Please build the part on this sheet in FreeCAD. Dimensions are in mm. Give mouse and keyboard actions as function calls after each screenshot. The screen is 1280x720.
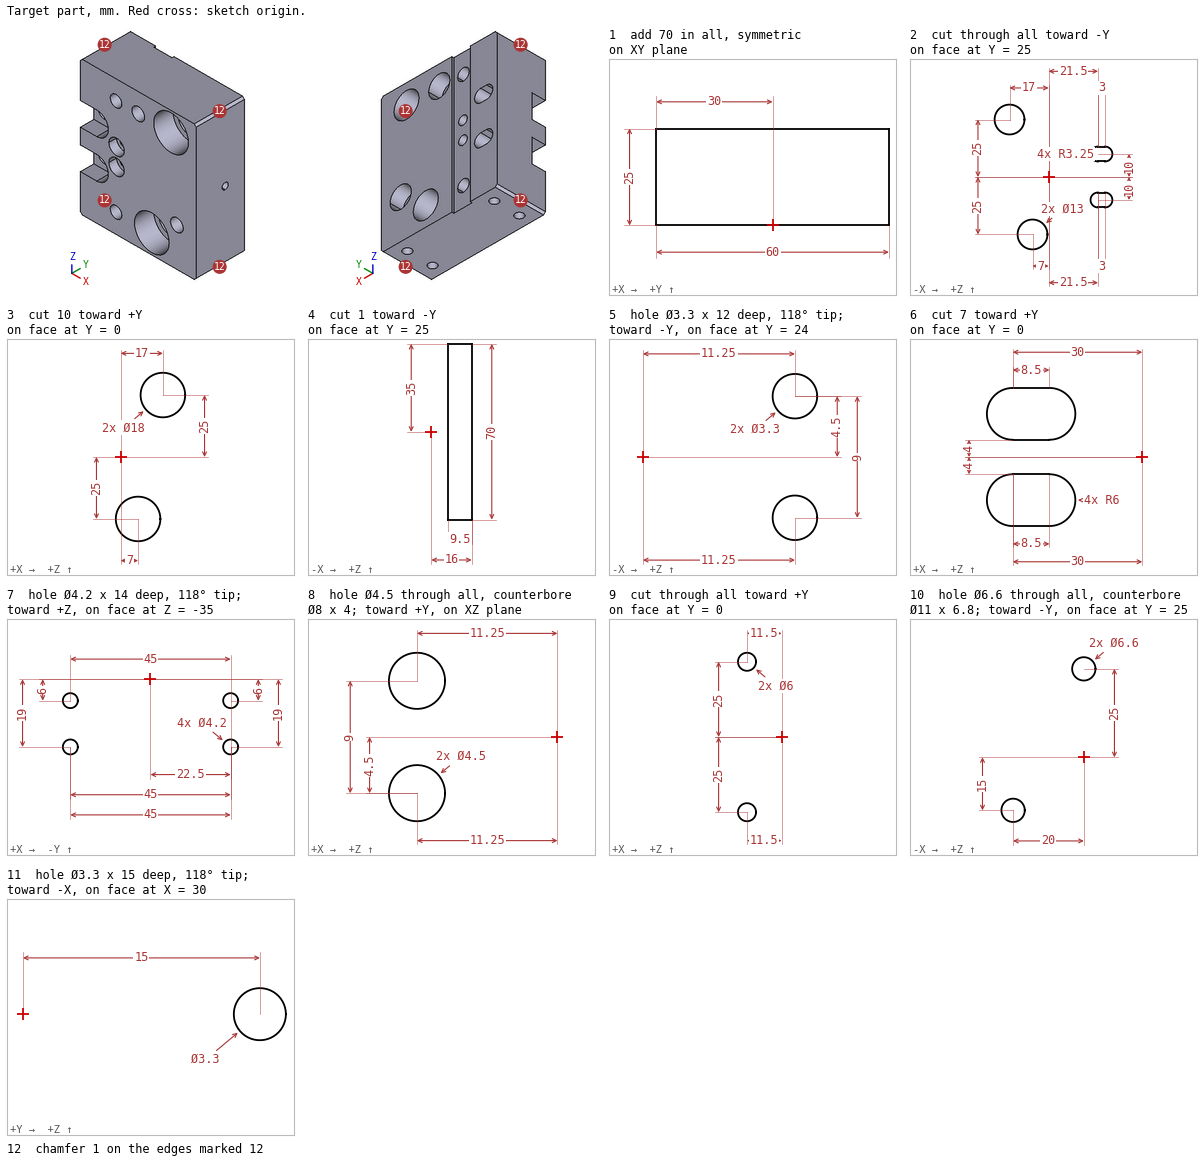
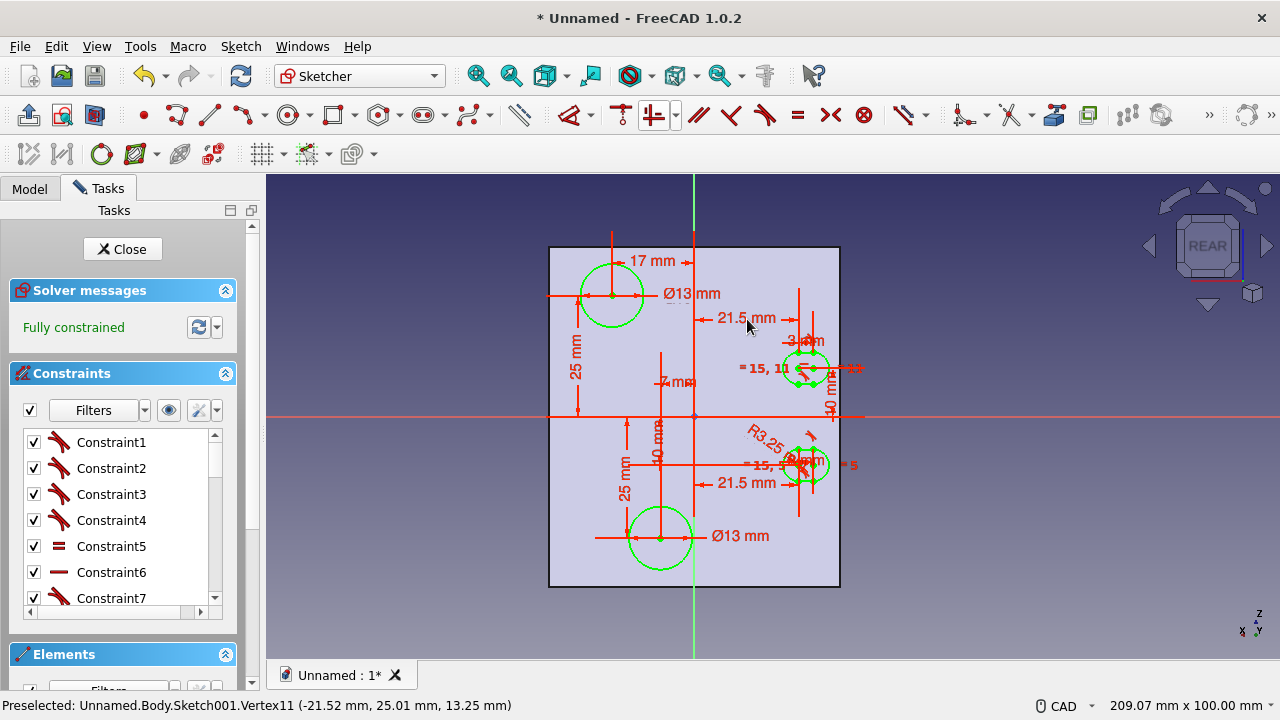
click(123, 249)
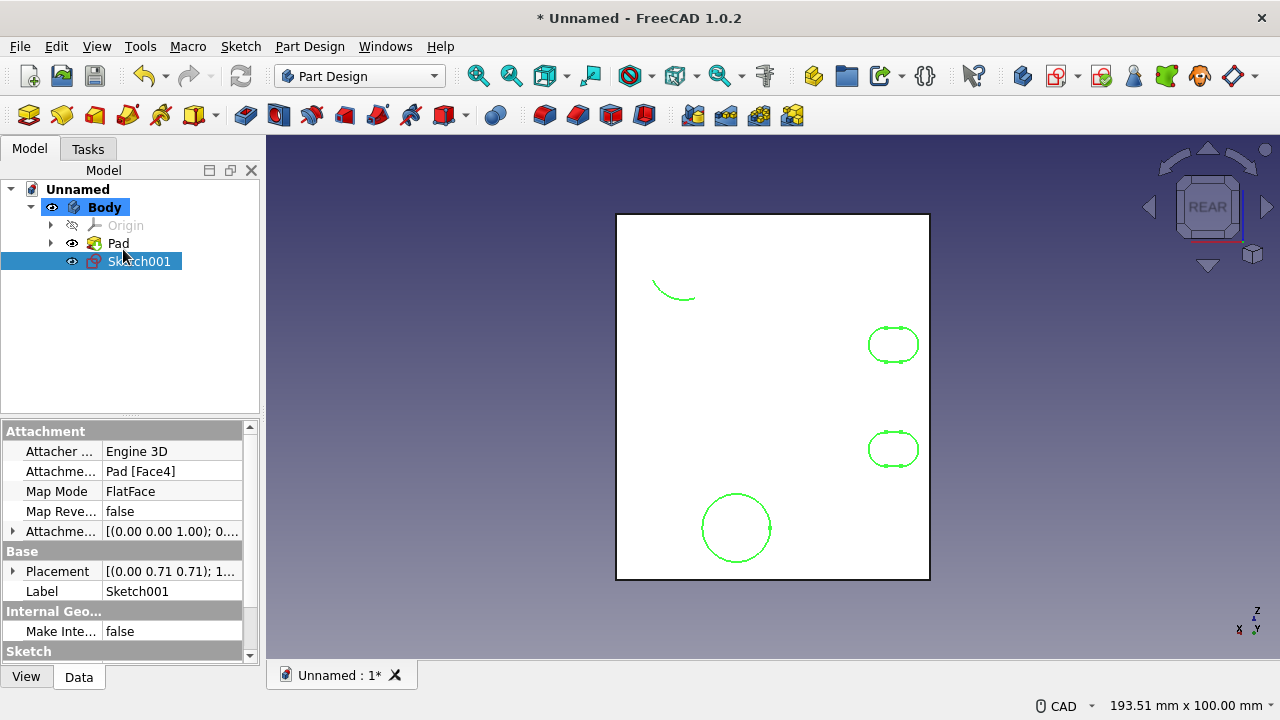
click(246, 116)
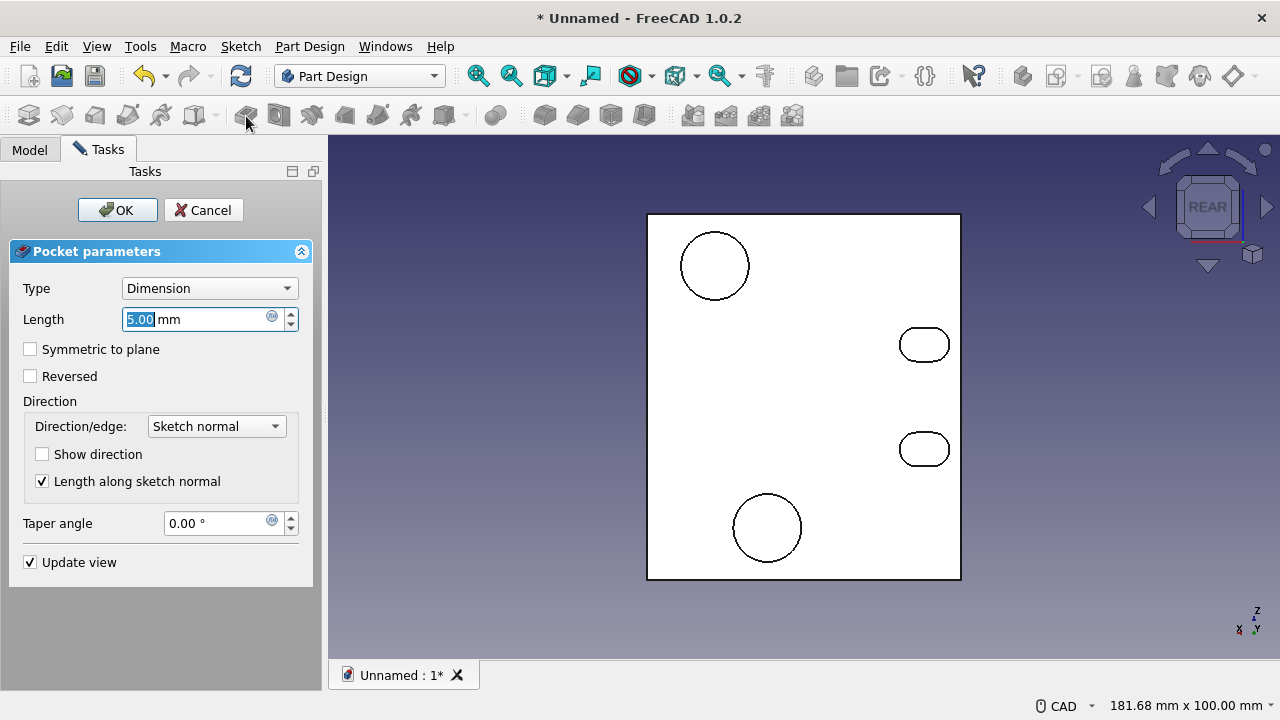
click(210, 288)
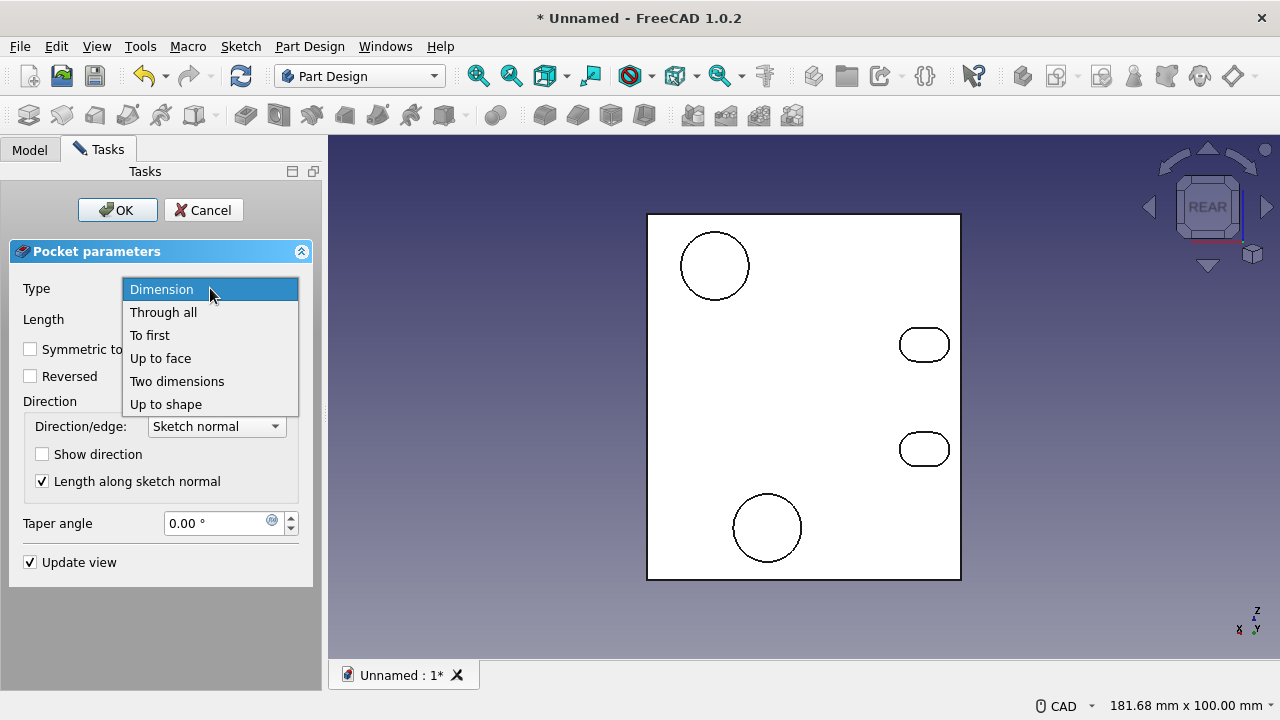
click(208, 312)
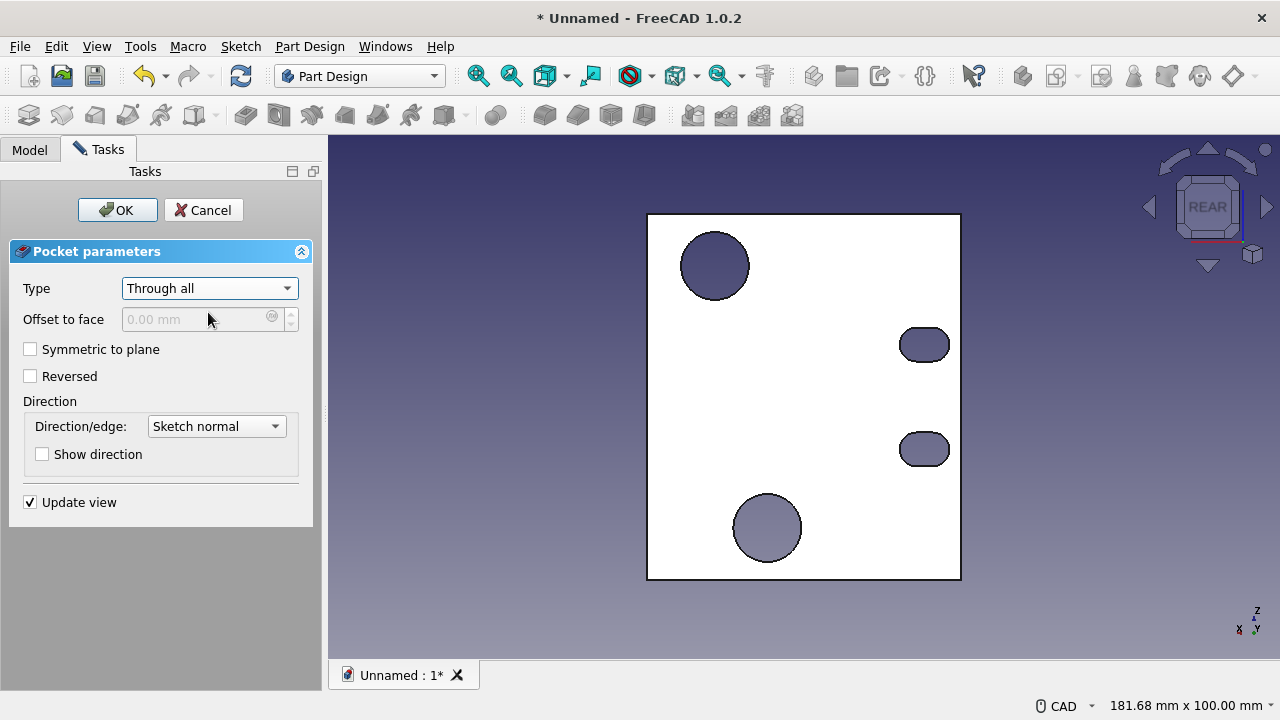
click(118, 210)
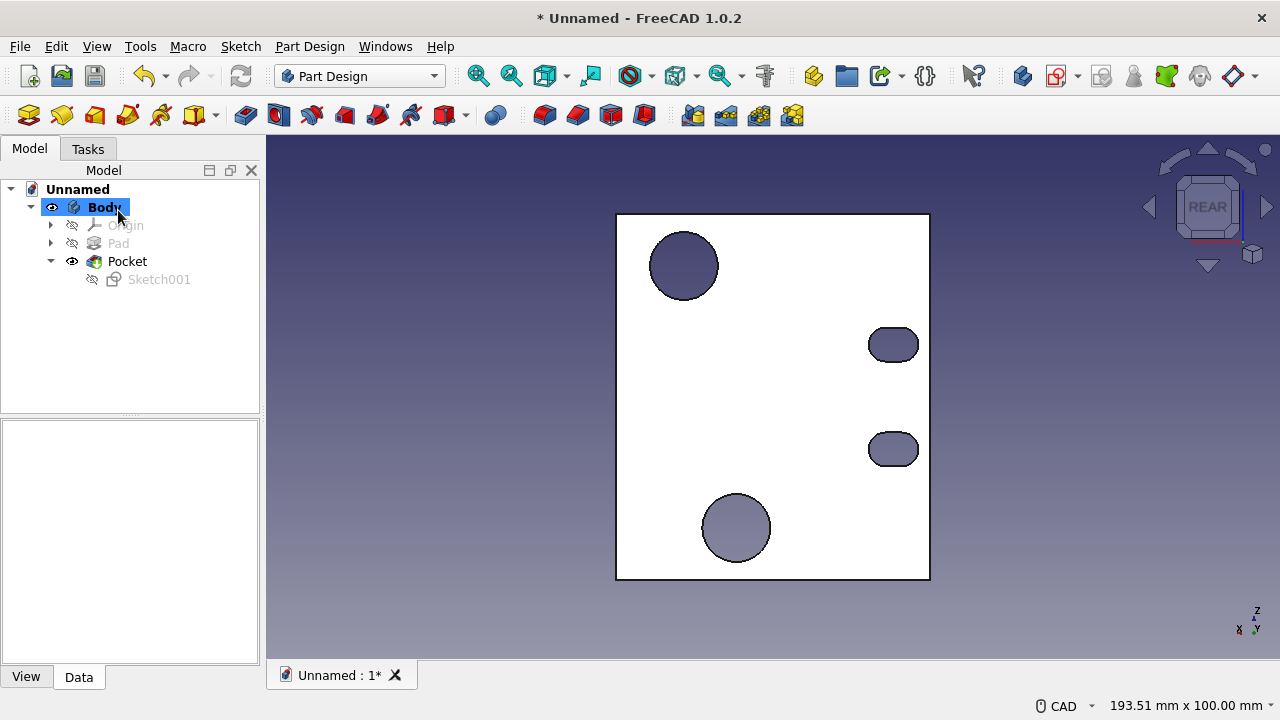
key(0)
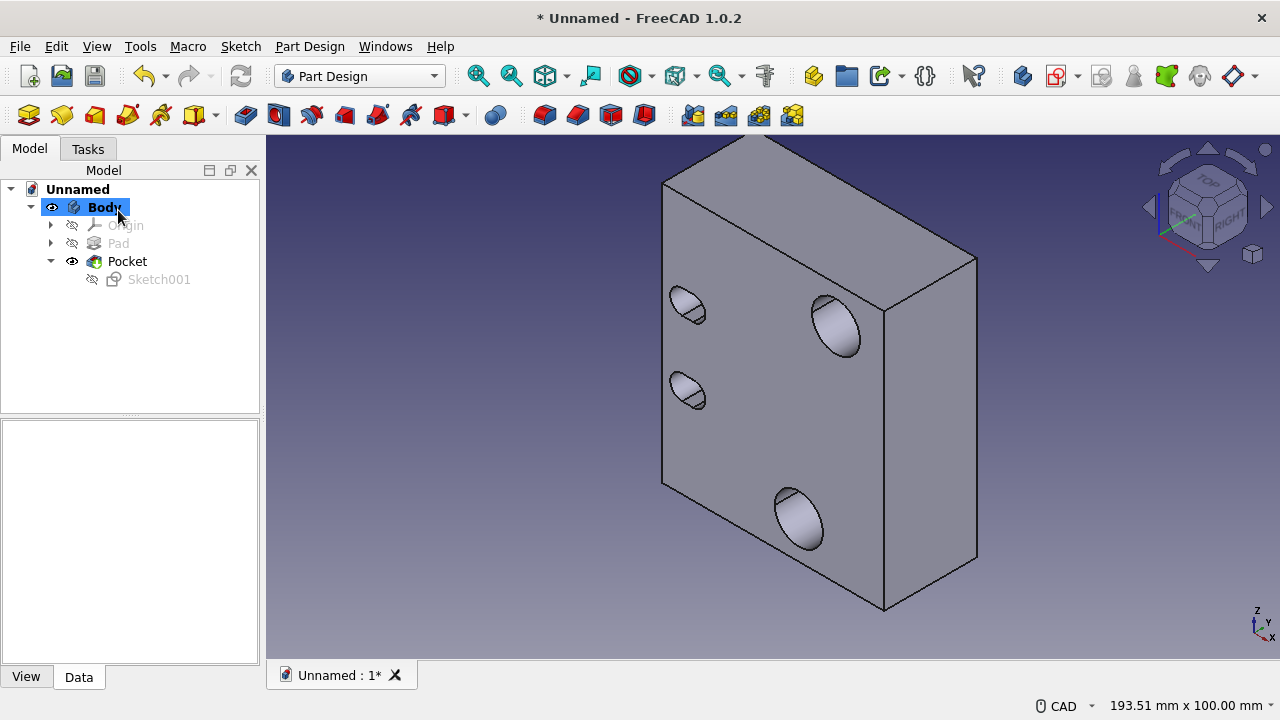
key(v)
key(f)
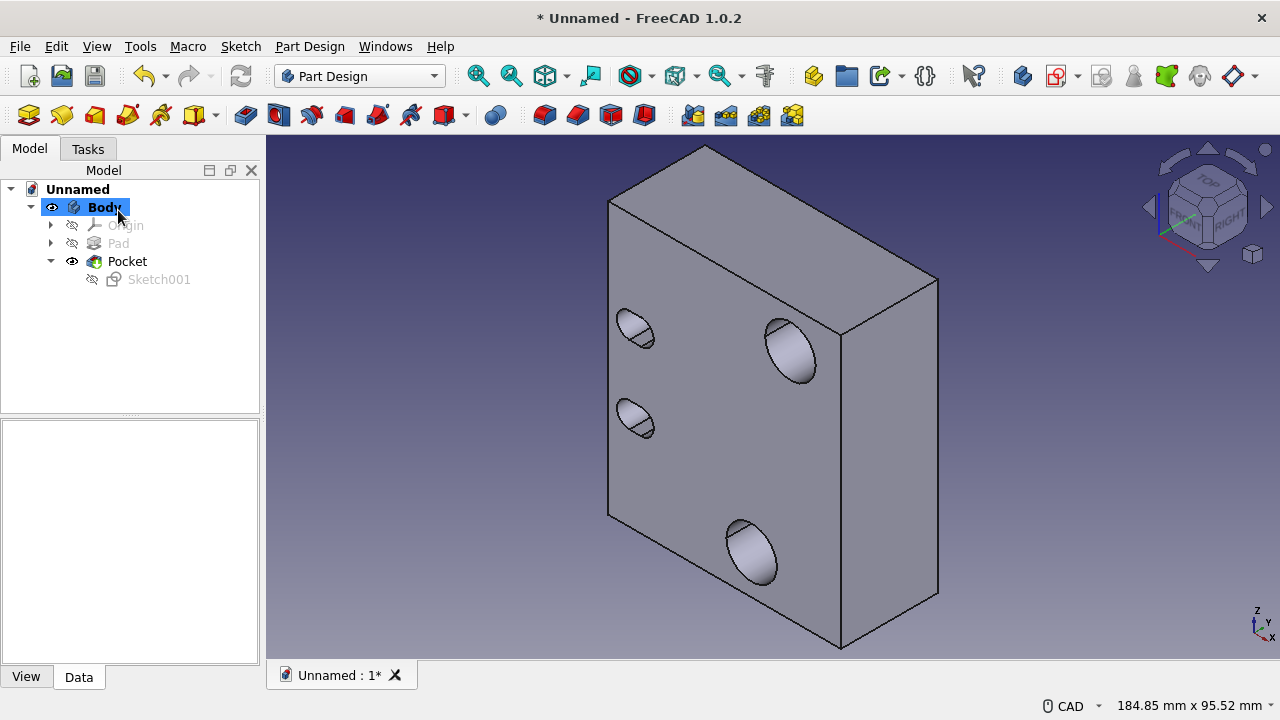
click(725, 424)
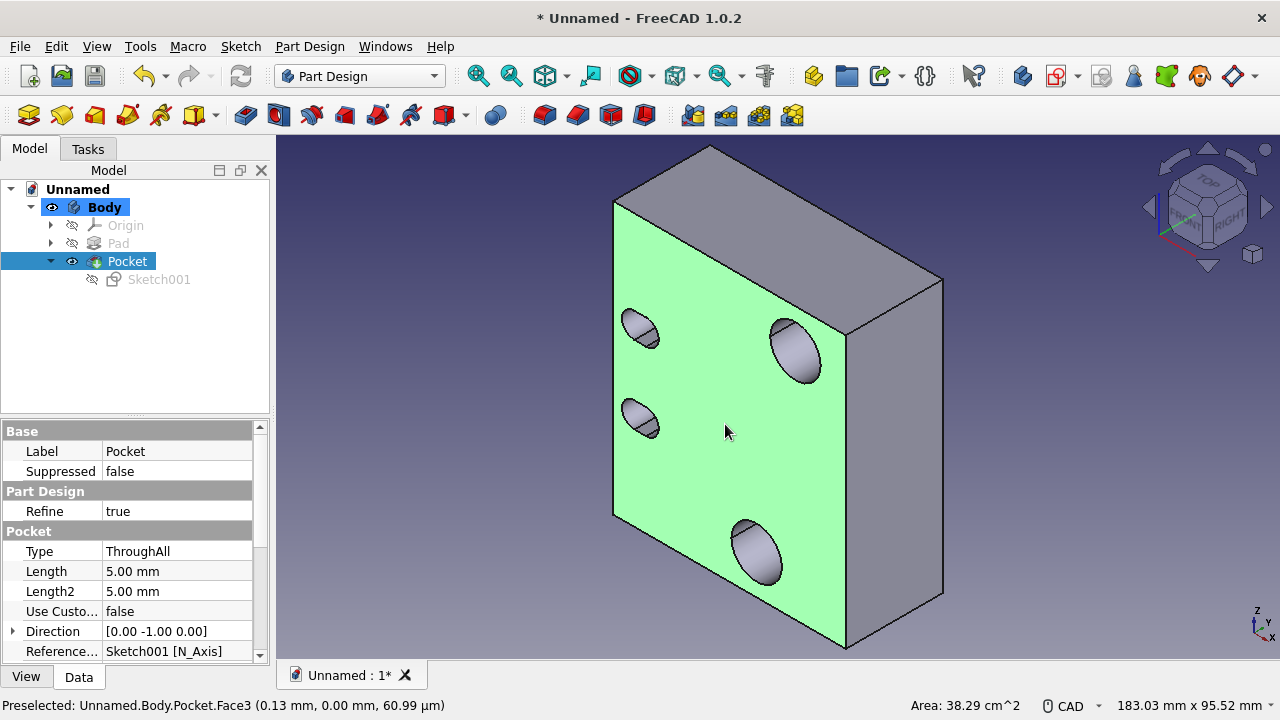
click(1056, 76)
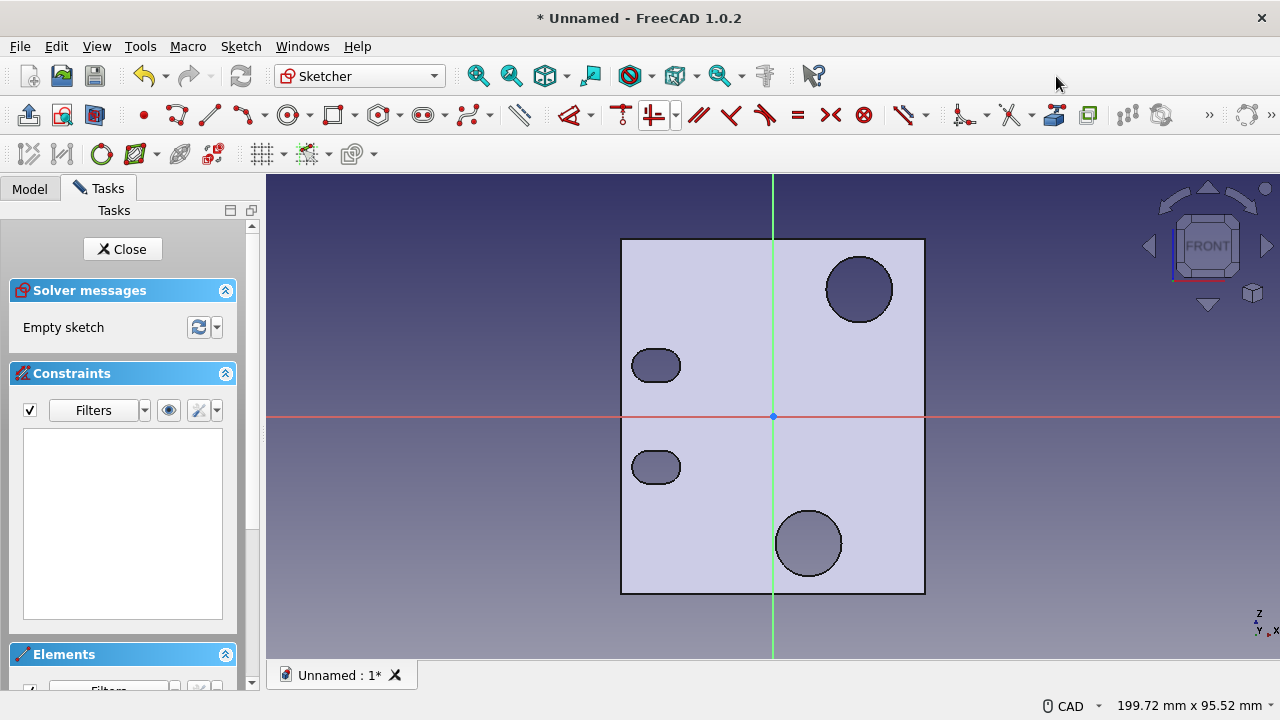
click(288, 116)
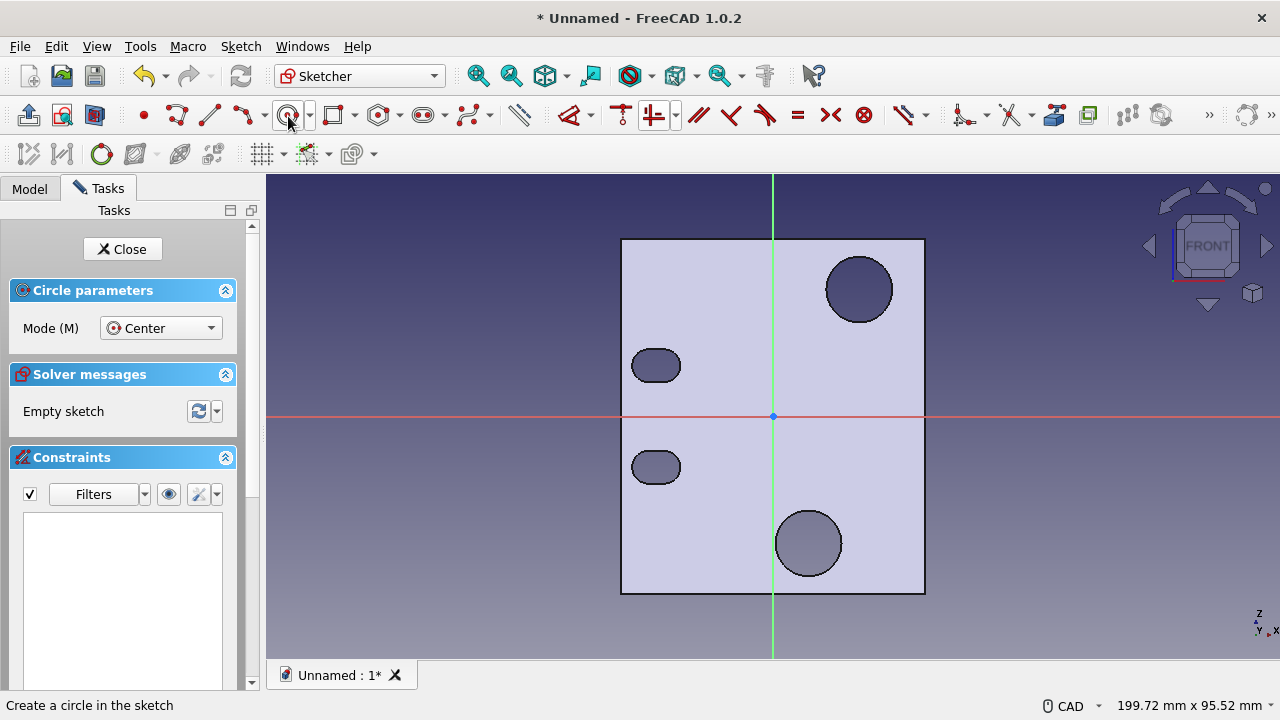
click(859, 290)
move(892, 257)